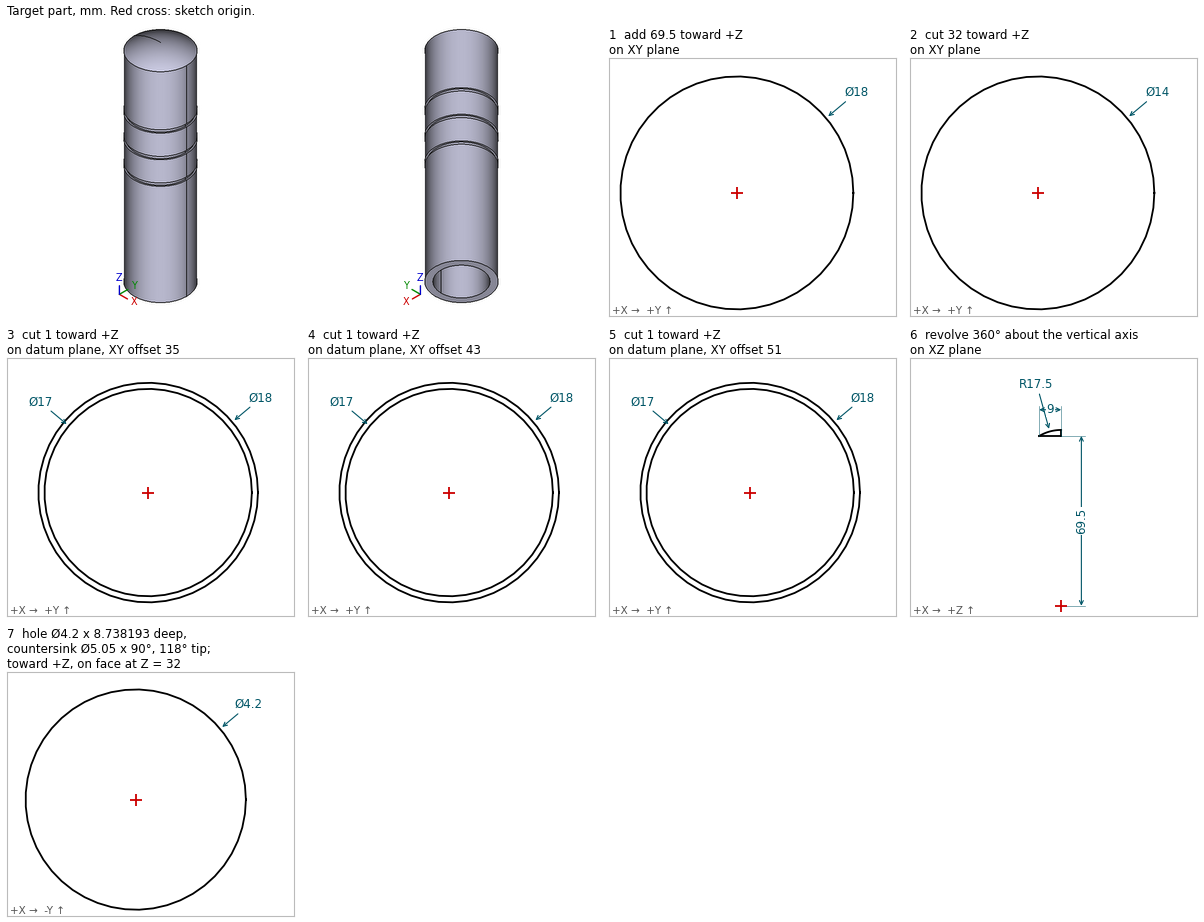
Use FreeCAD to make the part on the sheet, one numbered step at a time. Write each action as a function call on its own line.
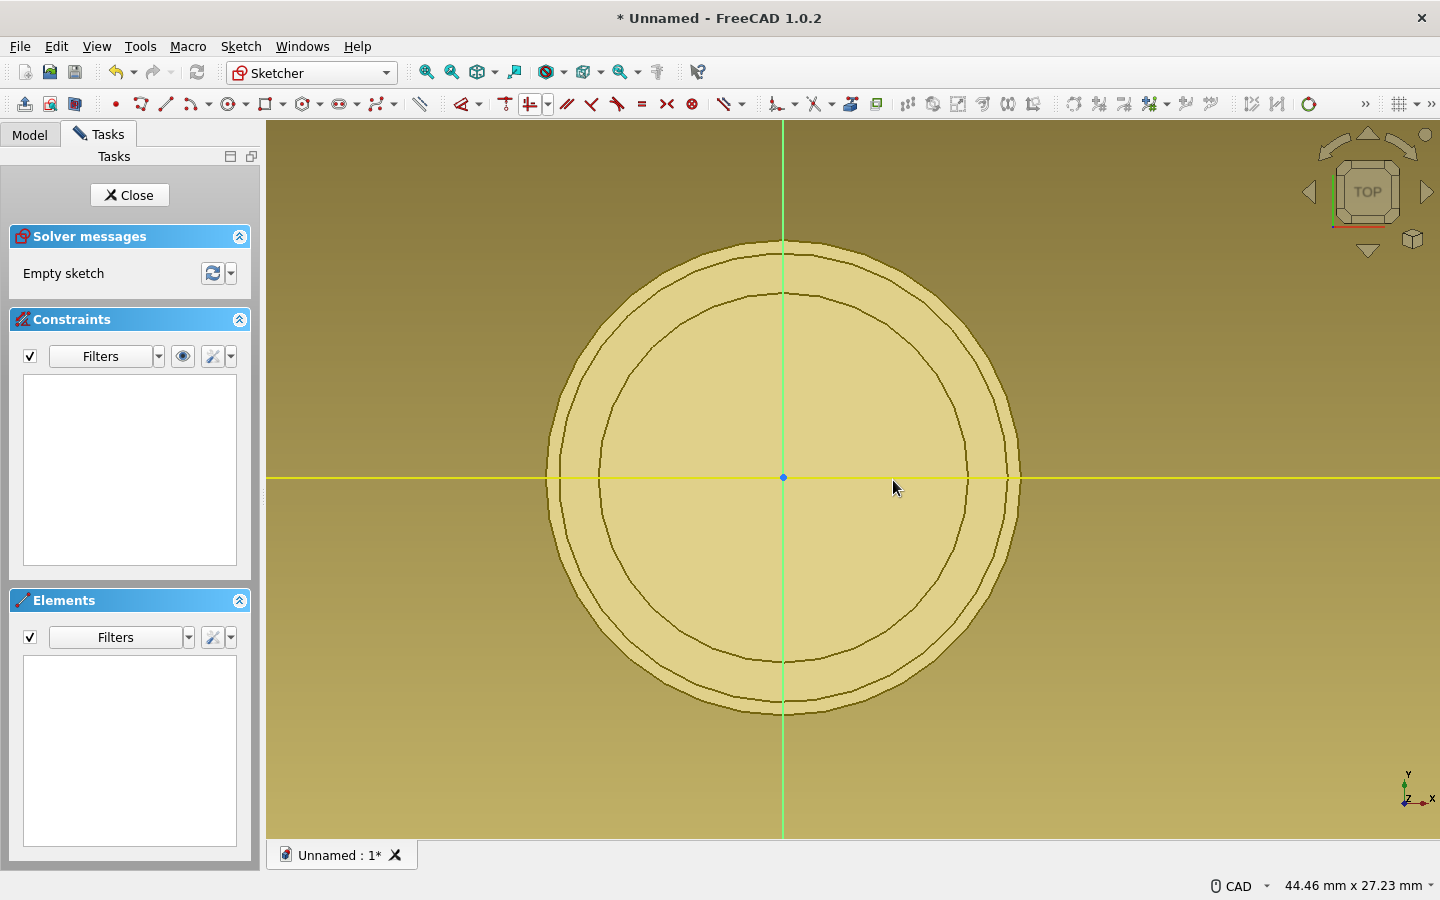
click(228, 104)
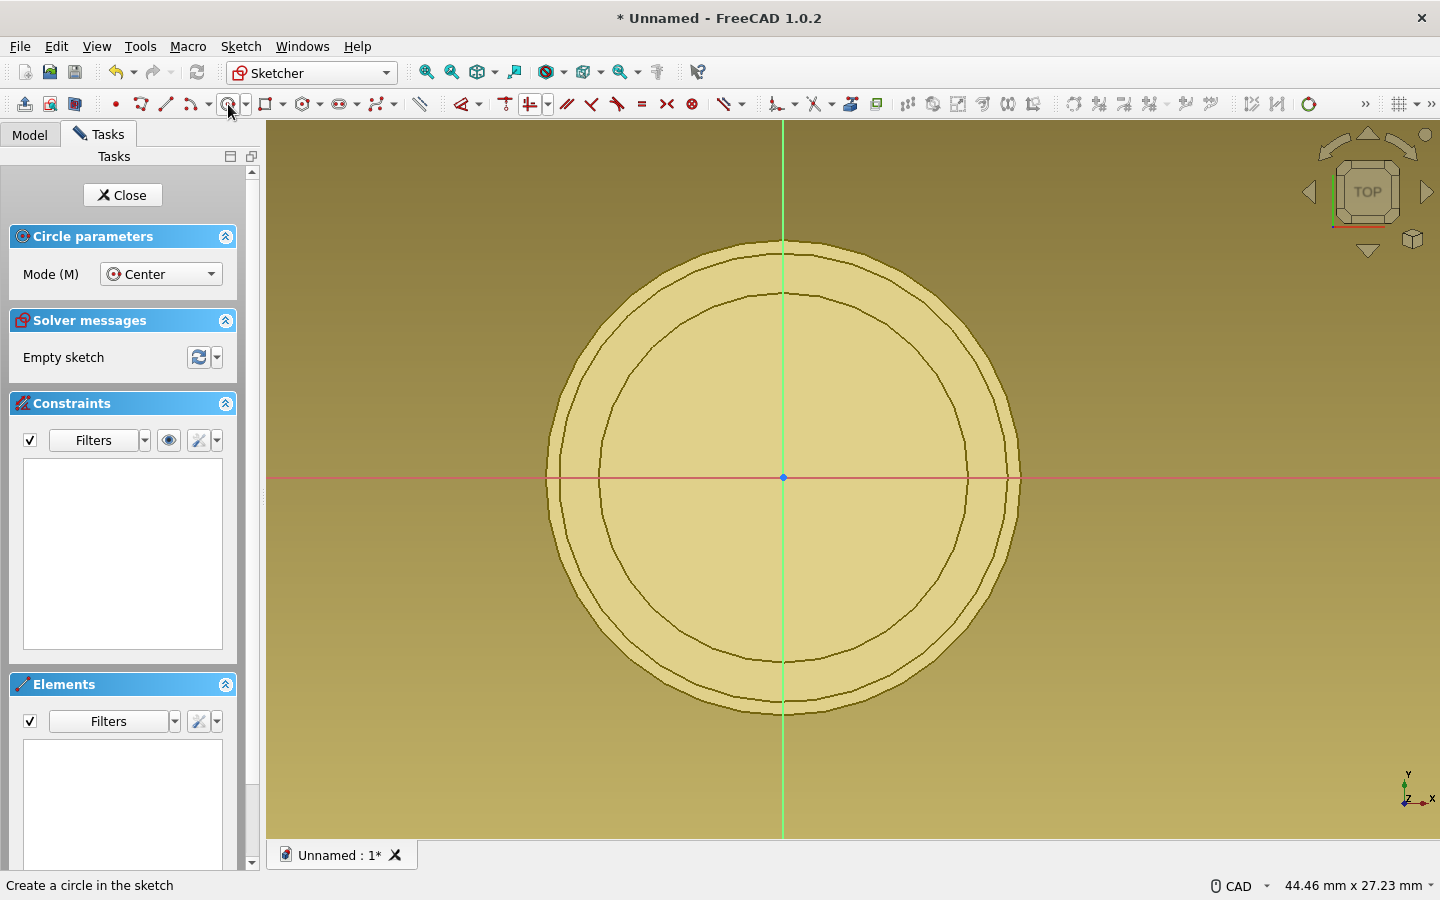
click(783, 478)
click(951, 310)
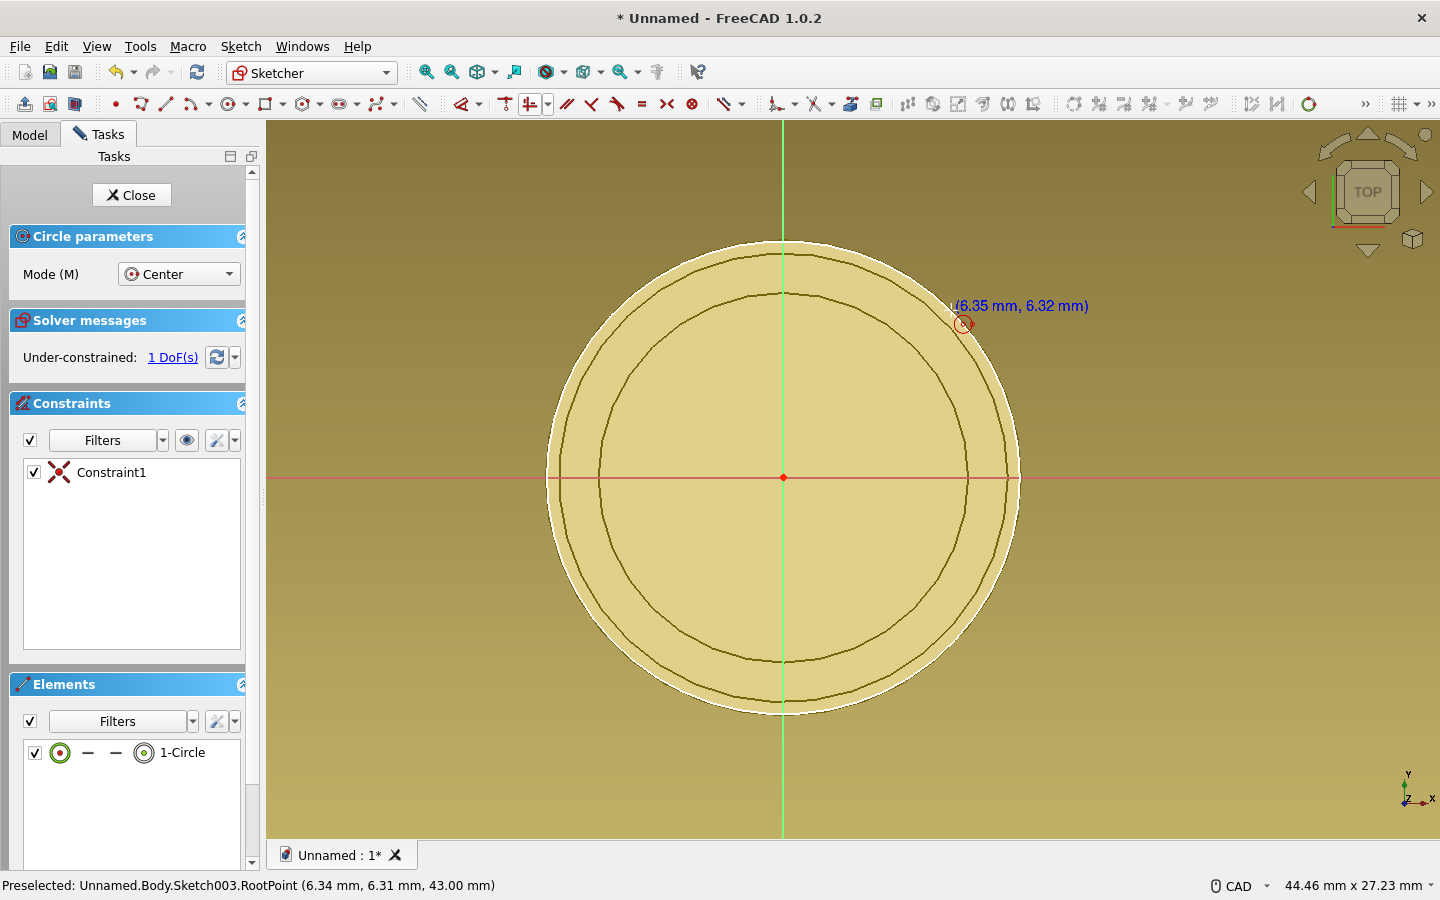
click(783, 478)
click(942, 319)
key(Escape)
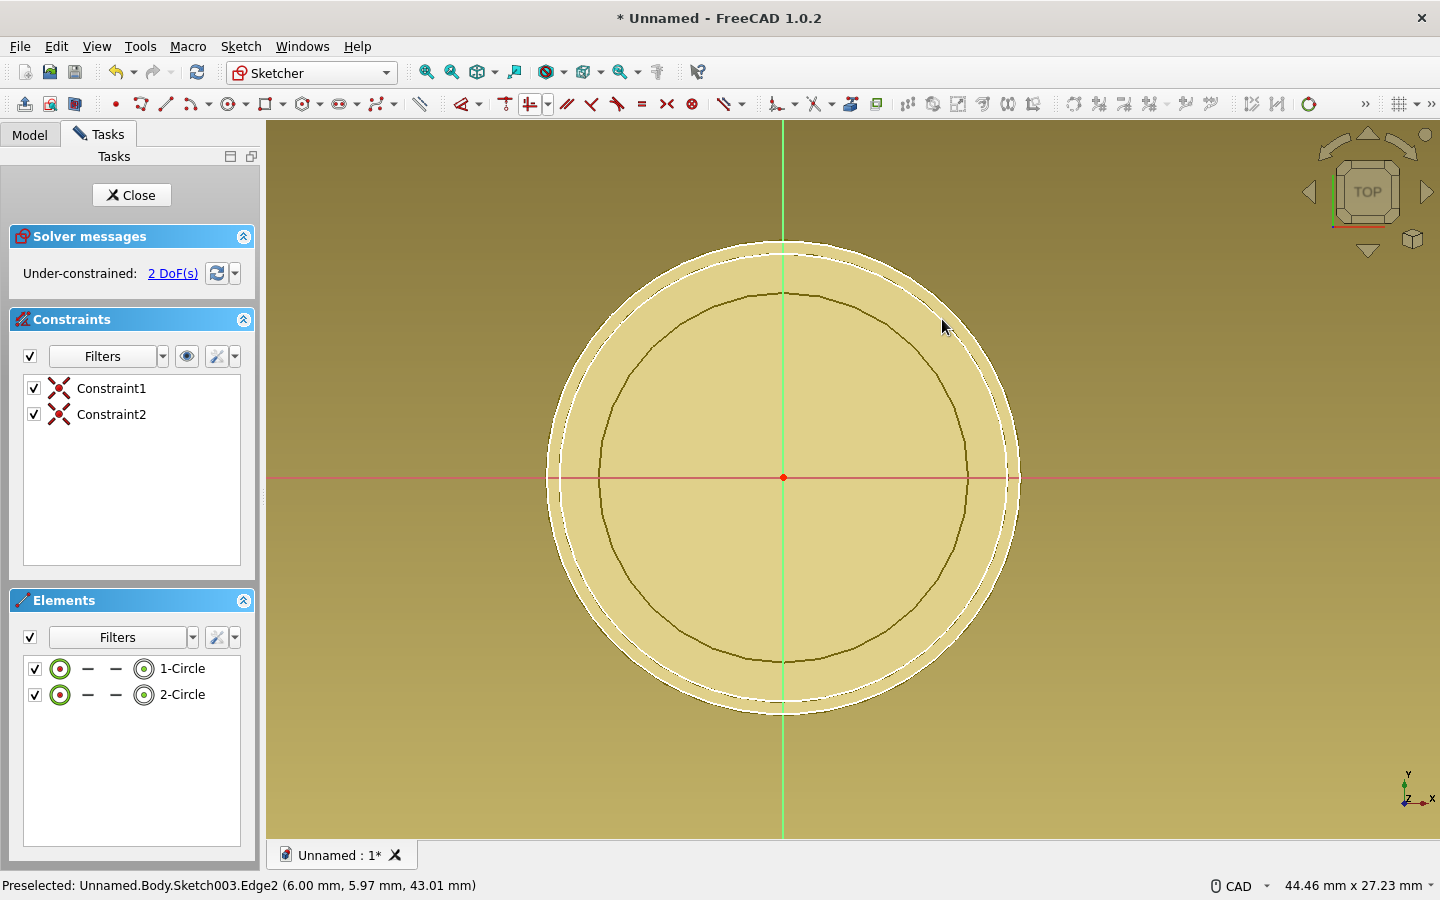
click(460, 104)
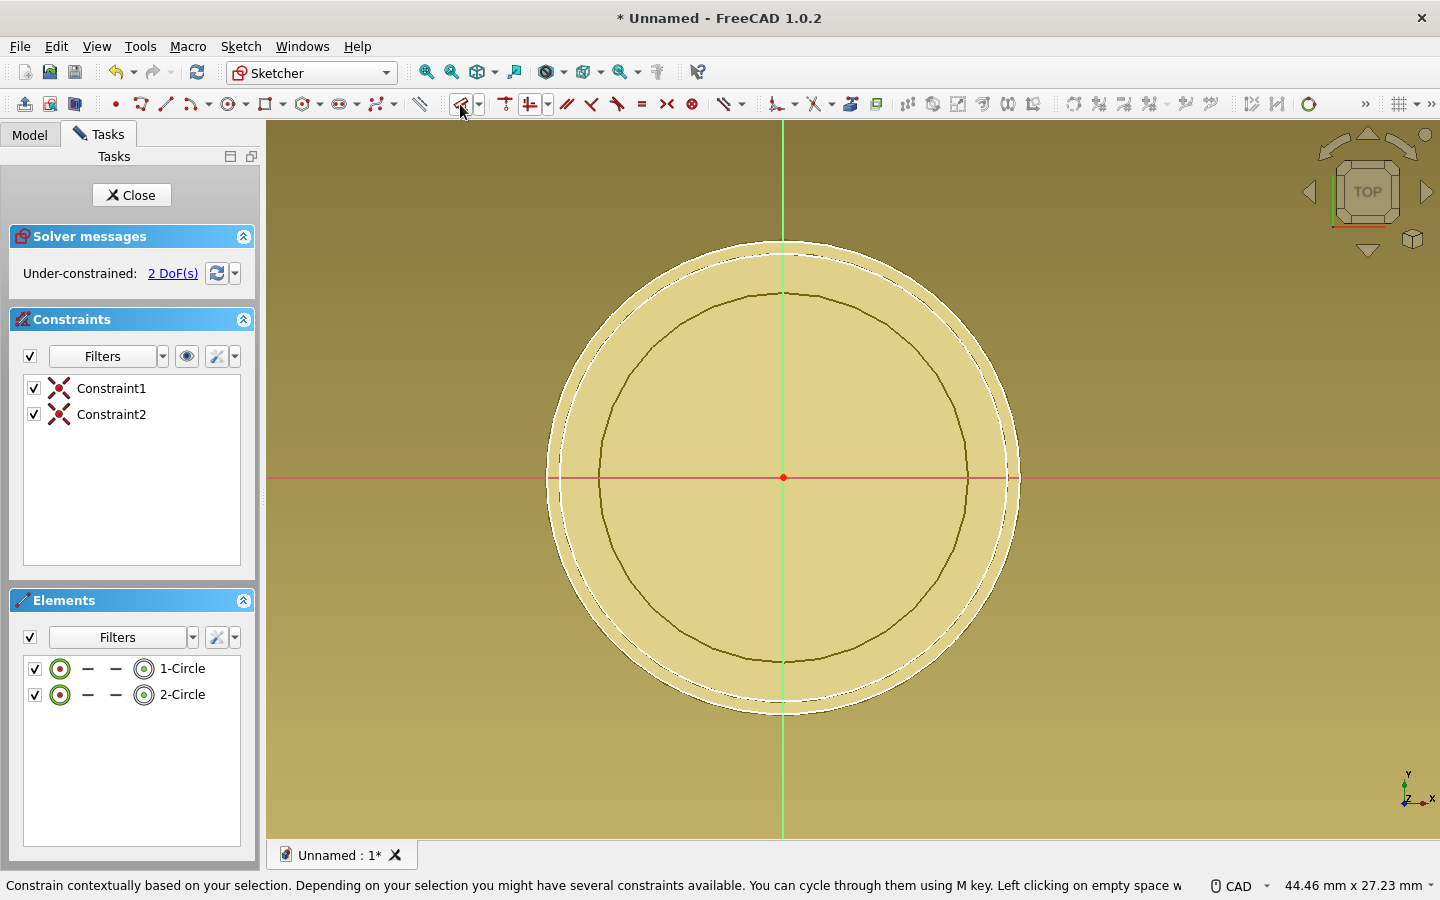
click(950, 310)
click(973, 287)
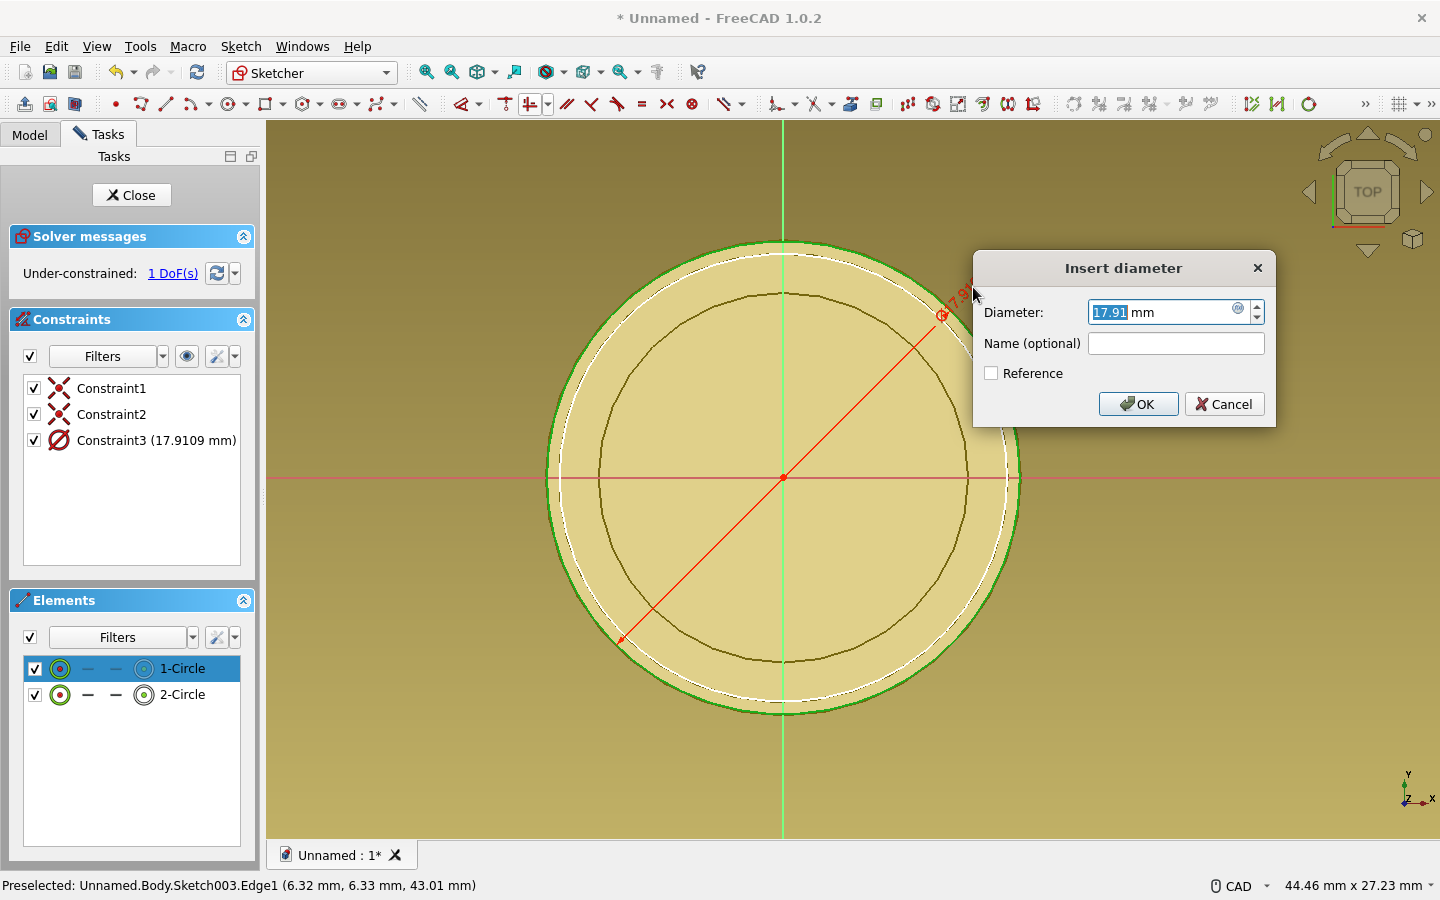
text(18)
key(Return)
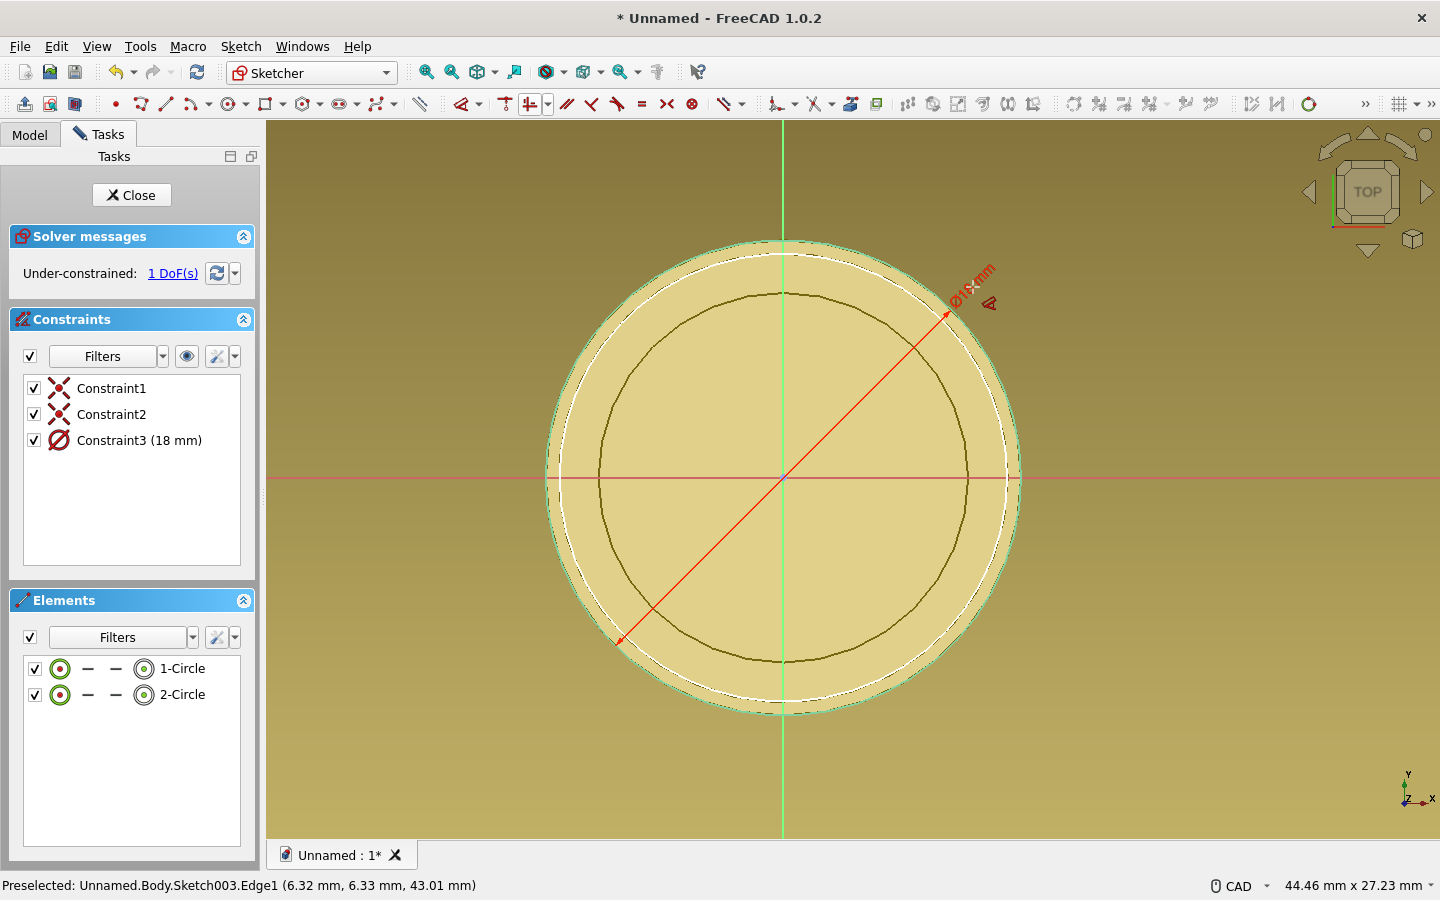
click(941, 319)
click(1028, 405)